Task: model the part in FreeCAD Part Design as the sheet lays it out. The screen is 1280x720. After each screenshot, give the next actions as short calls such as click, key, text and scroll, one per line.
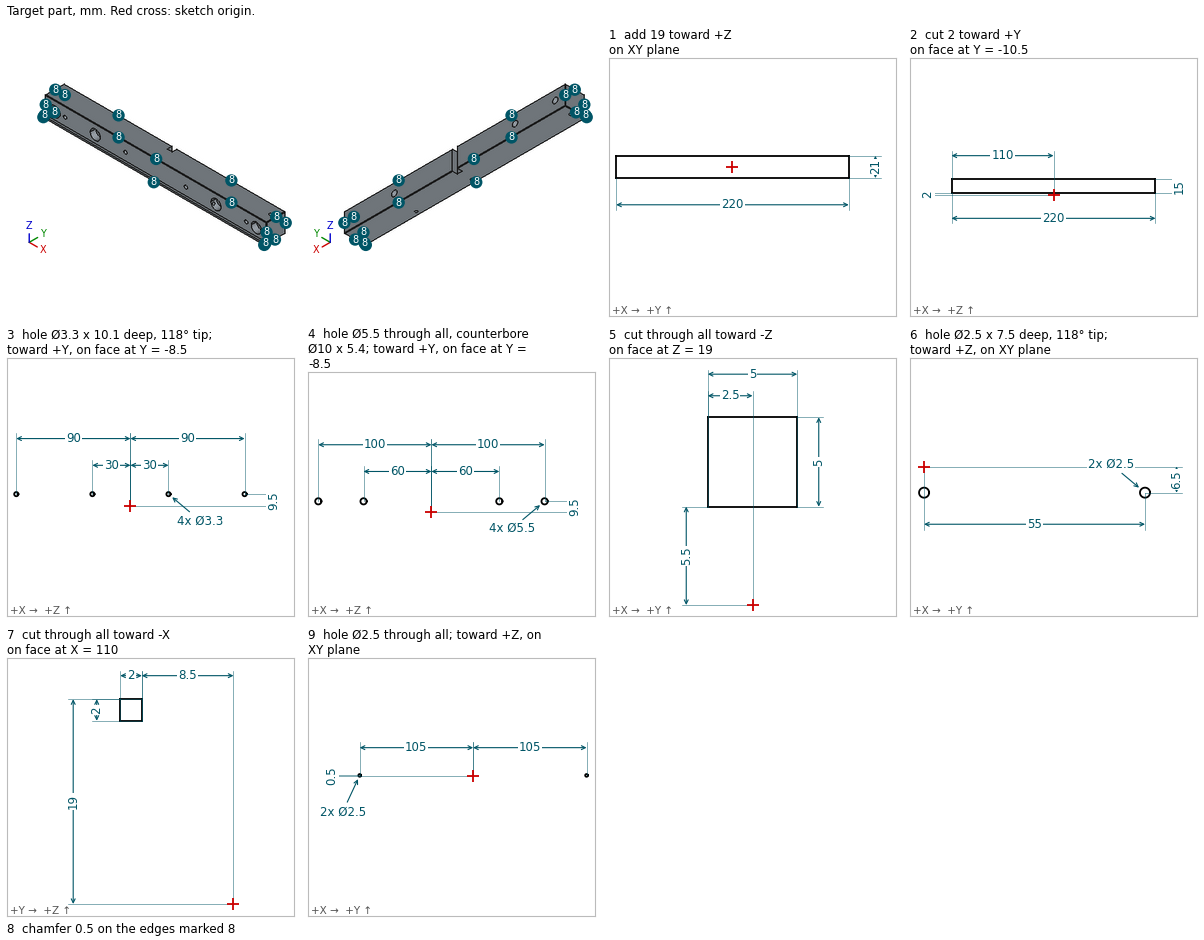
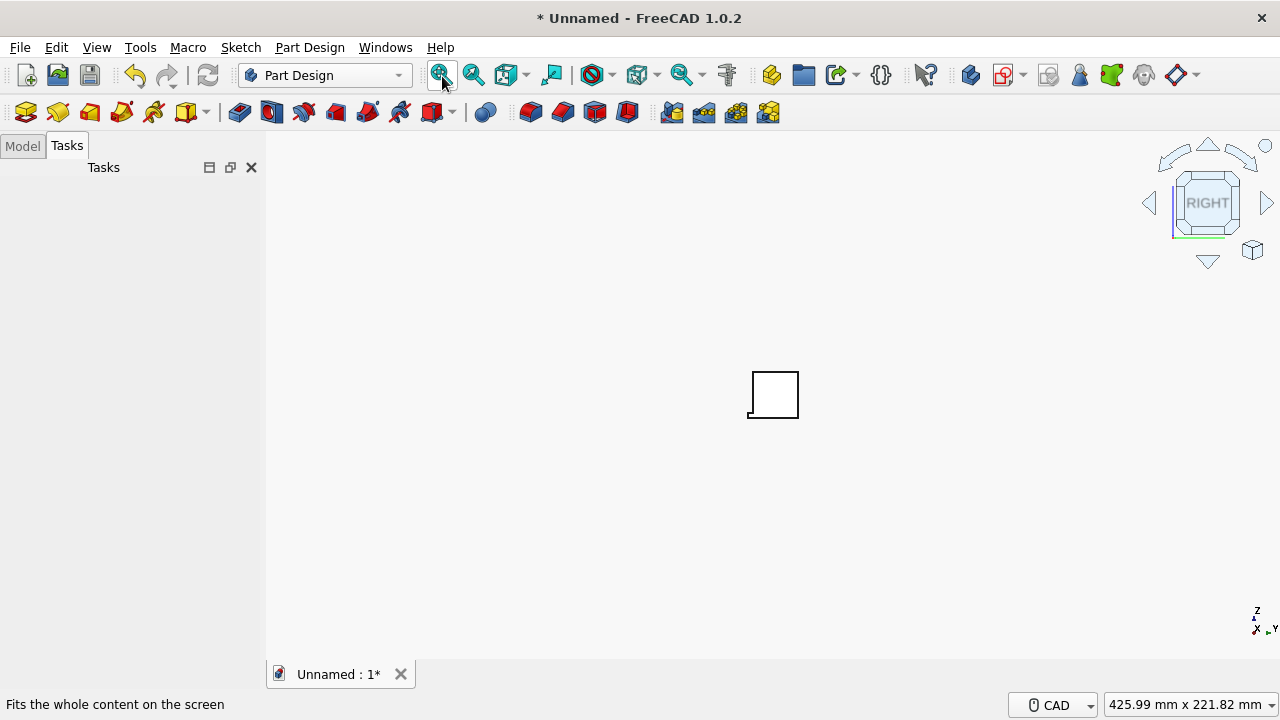
key(5)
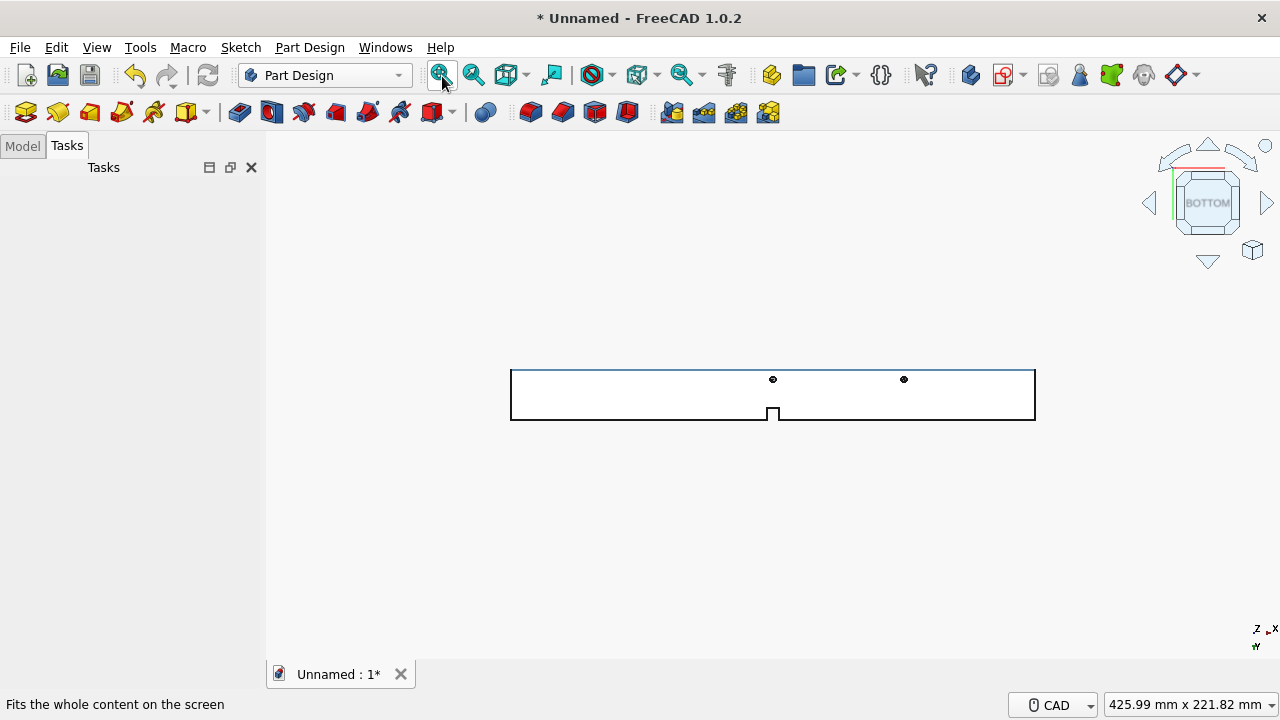
click(907, 419, ctrl)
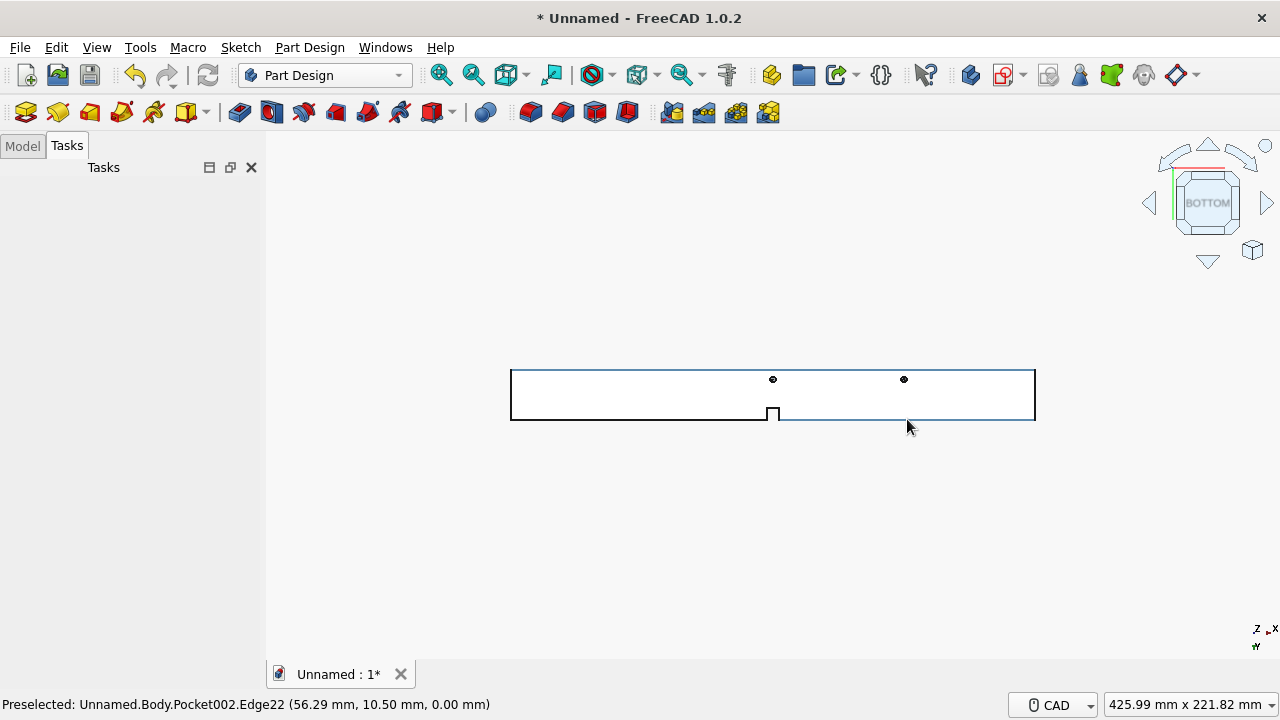
click(639, 419, ctrl)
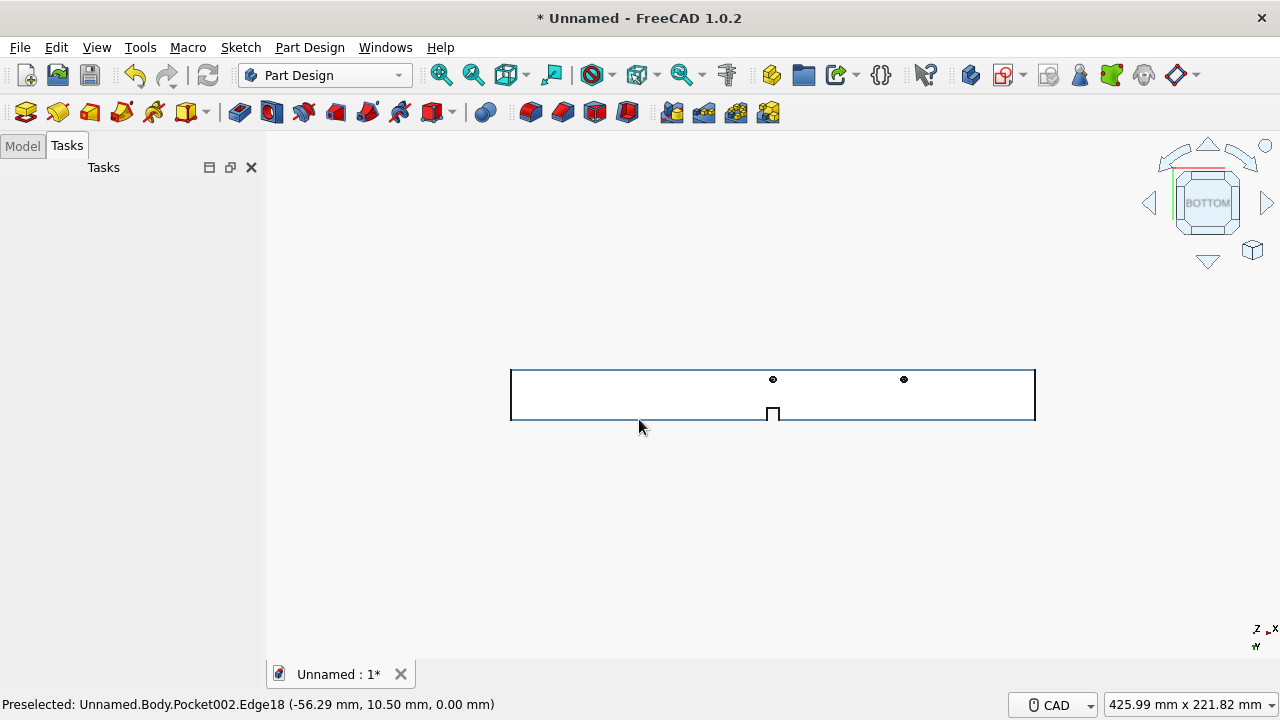
key(4)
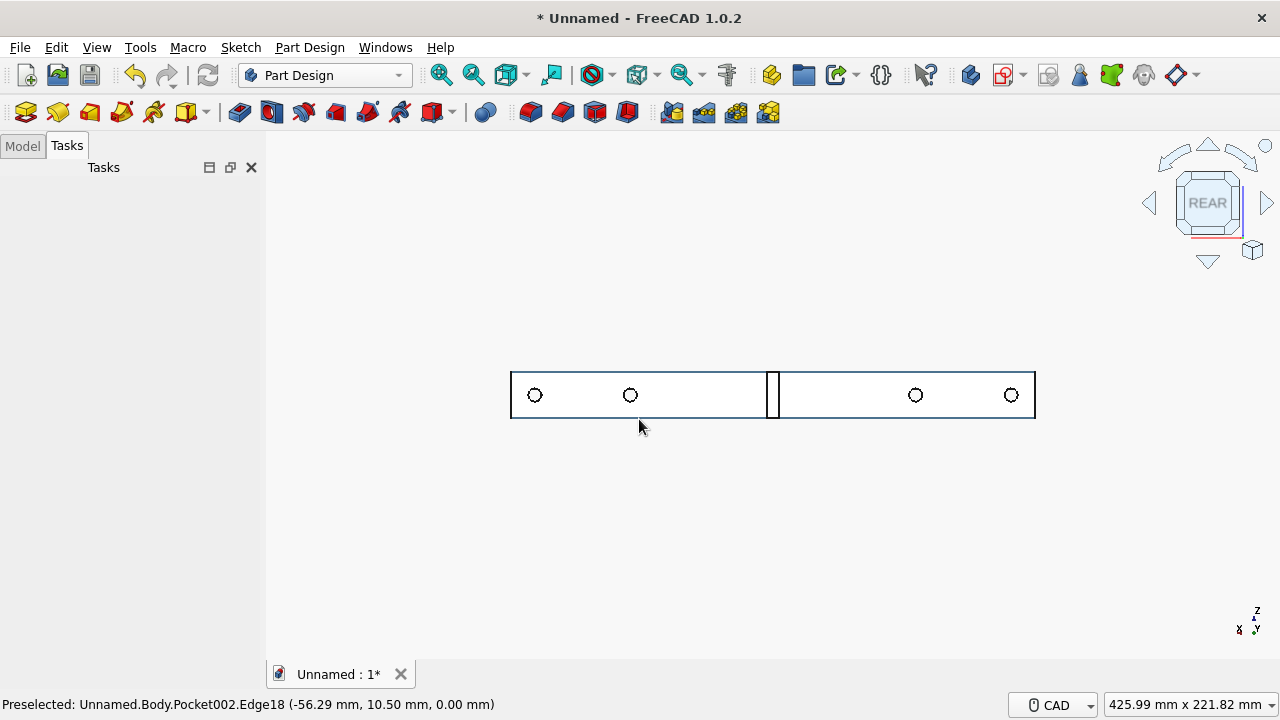
key(6)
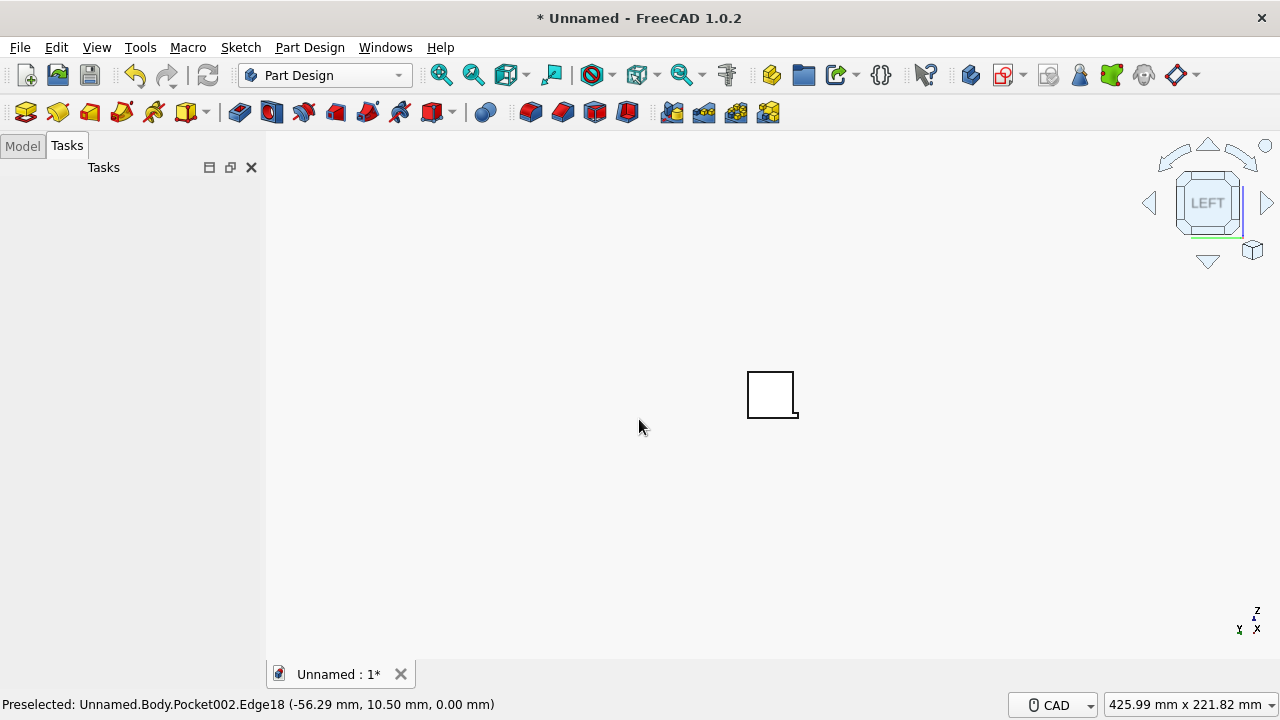
click(442, 76)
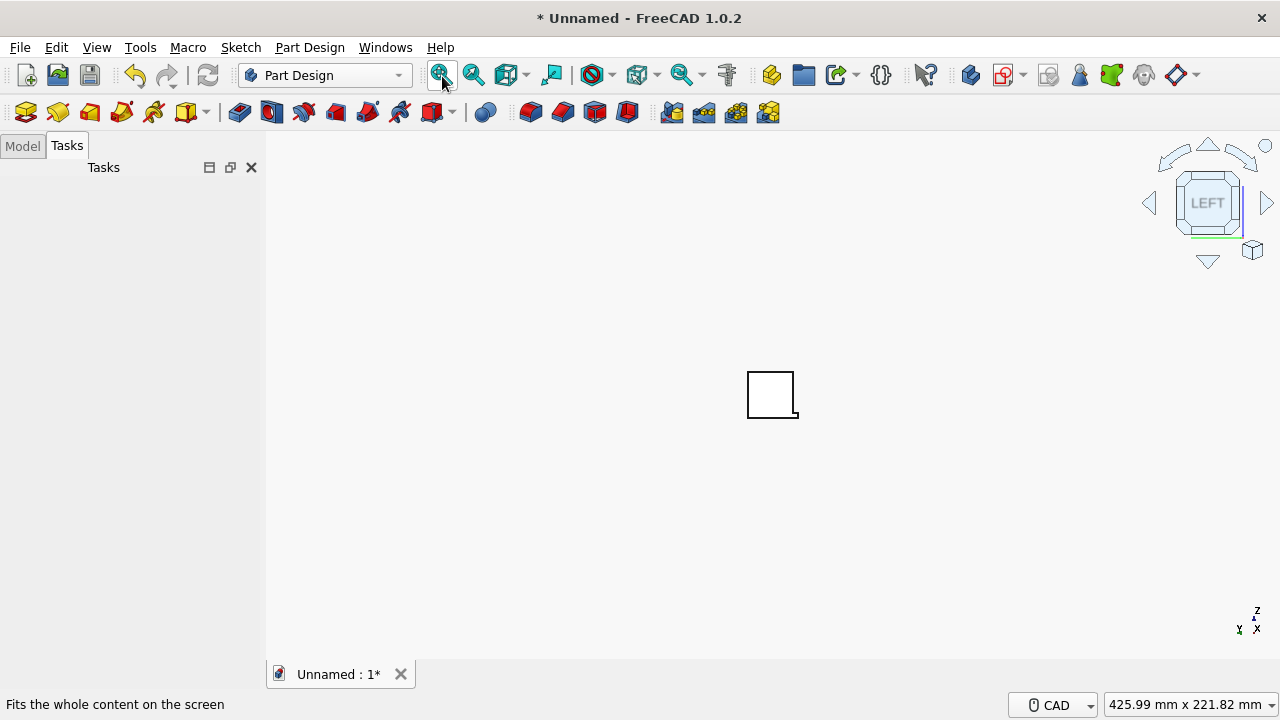
click(773, 394, ctrl)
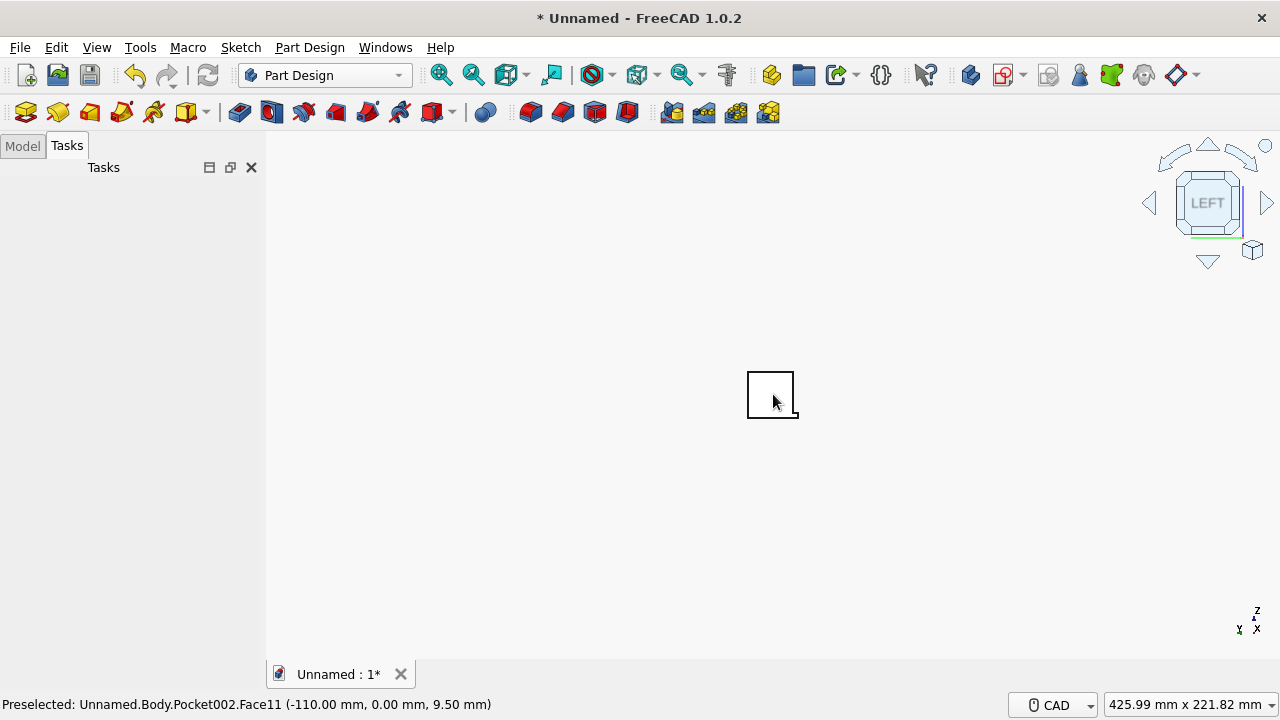
click(564, 112)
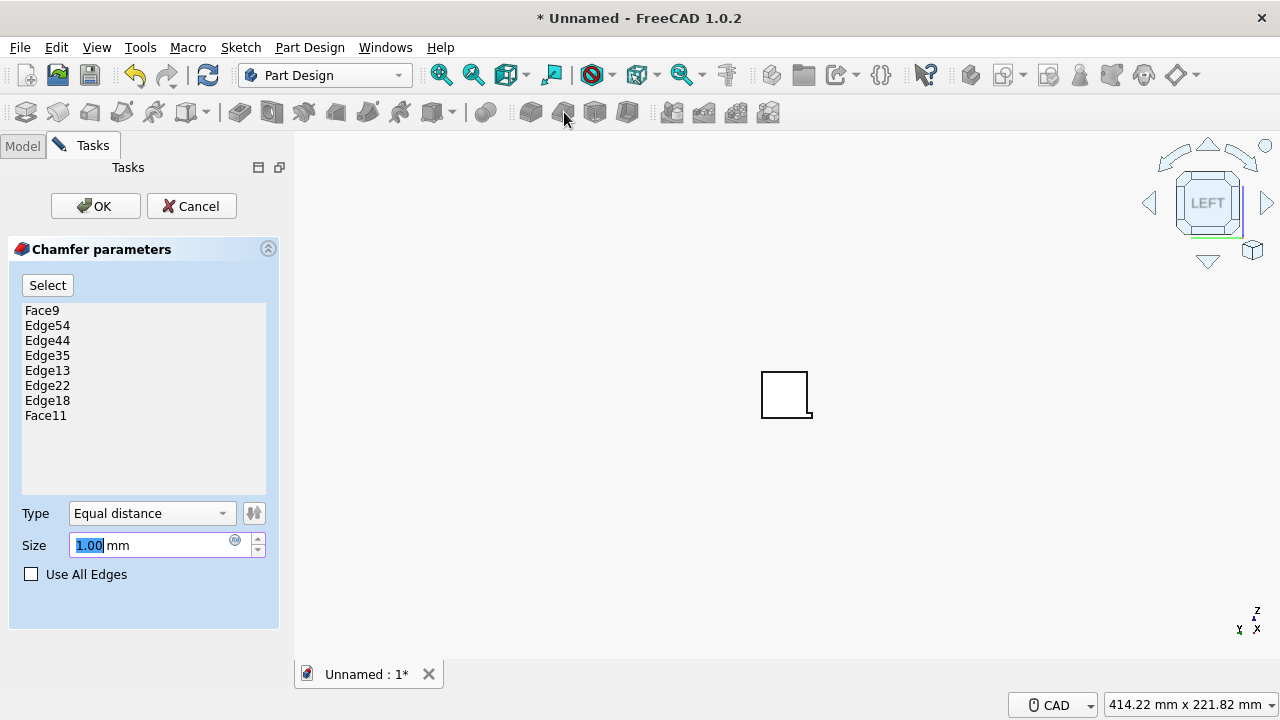
text(0.5)
key(Tab)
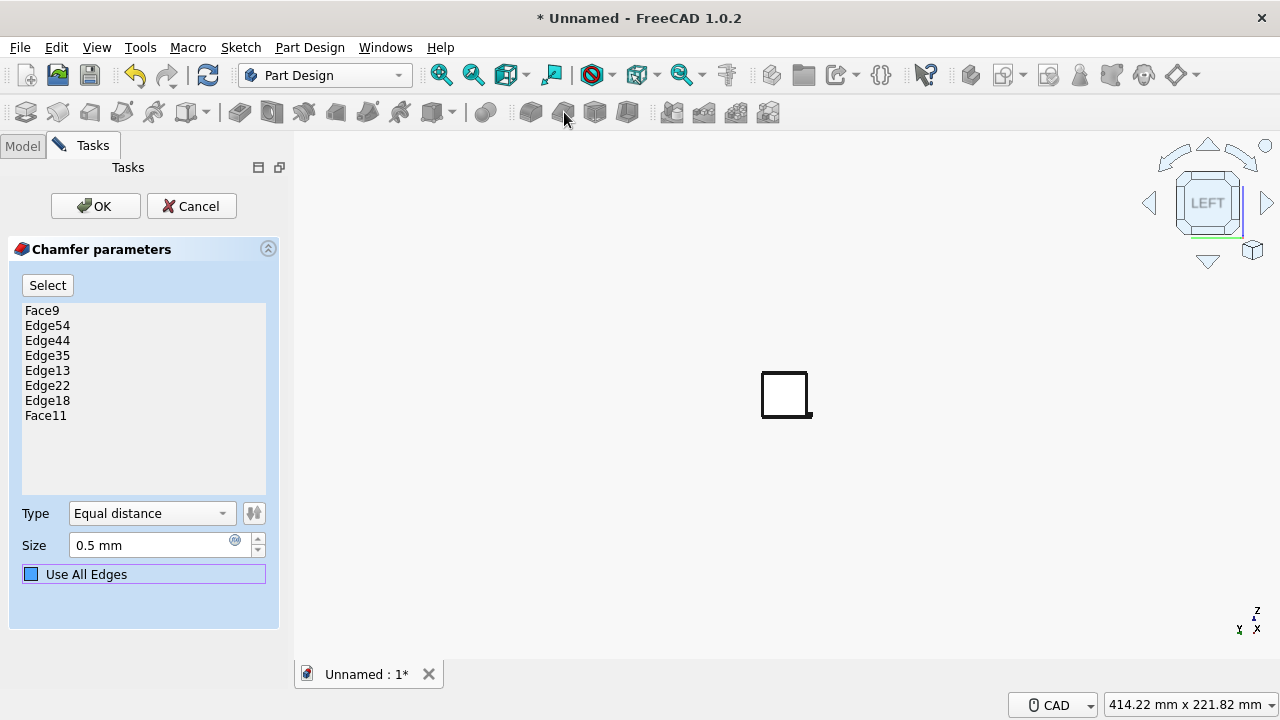
click(96, 206)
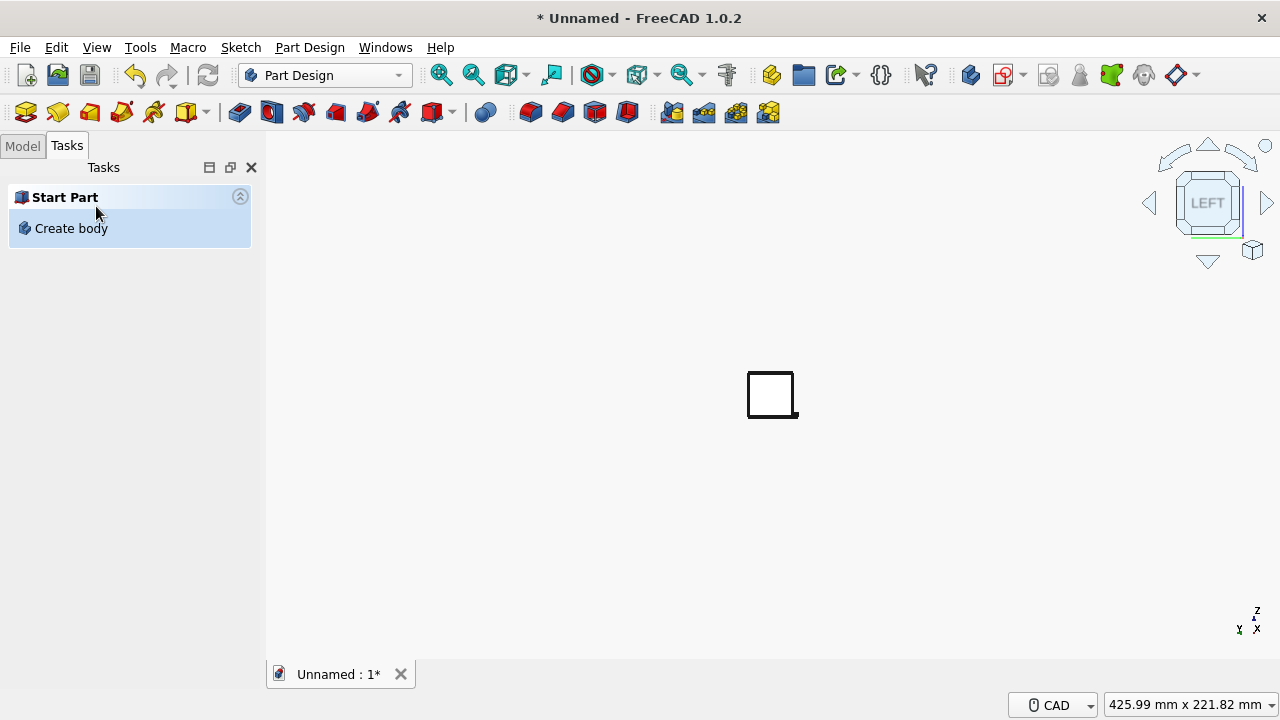
click(442, 76)